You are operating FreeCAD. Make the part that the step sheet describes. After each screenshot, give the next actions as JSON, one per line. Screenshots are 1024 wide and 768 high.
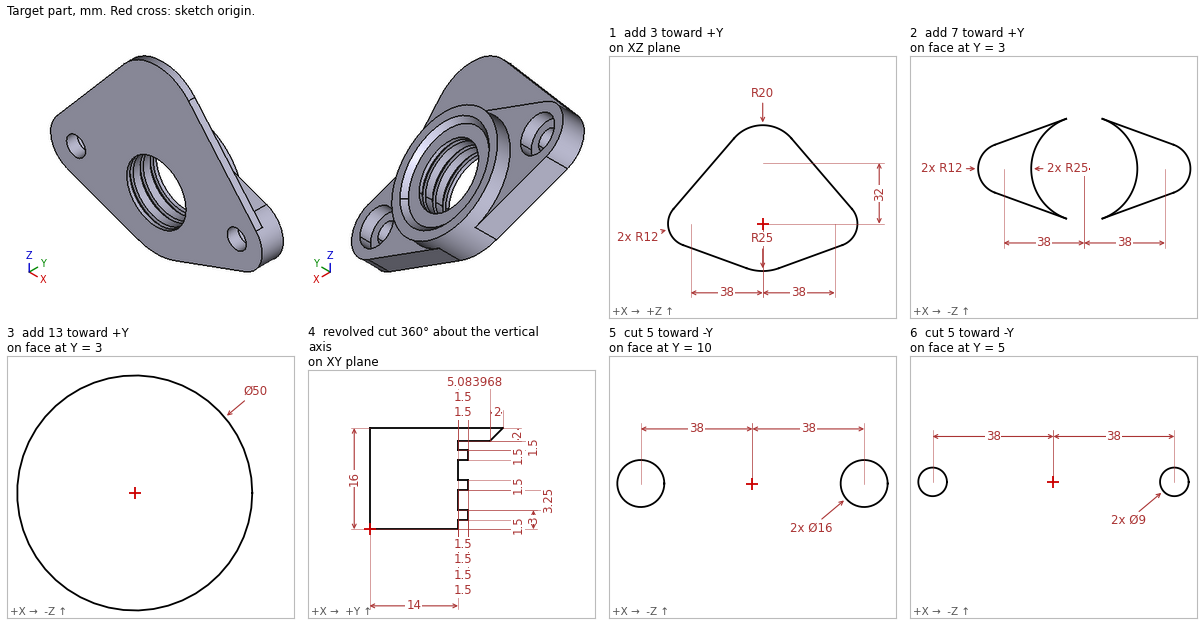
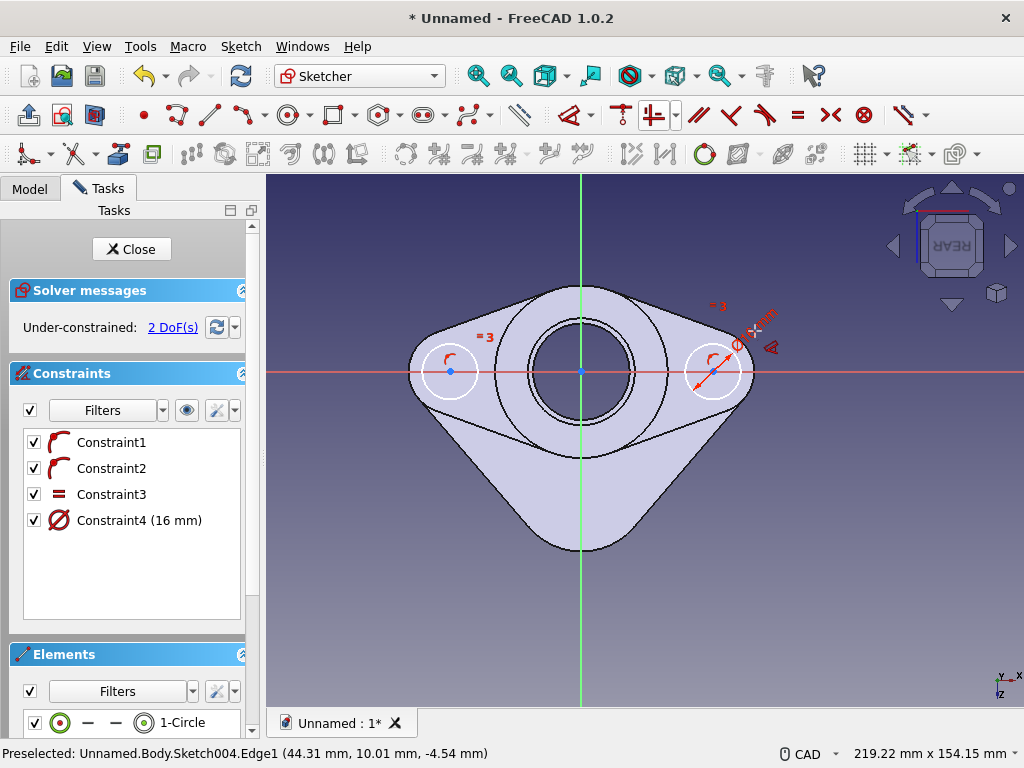
{"action": "left_click", "coordinate": [713, 372]}
{"action": "left_click", "coordinate": [647, 406]}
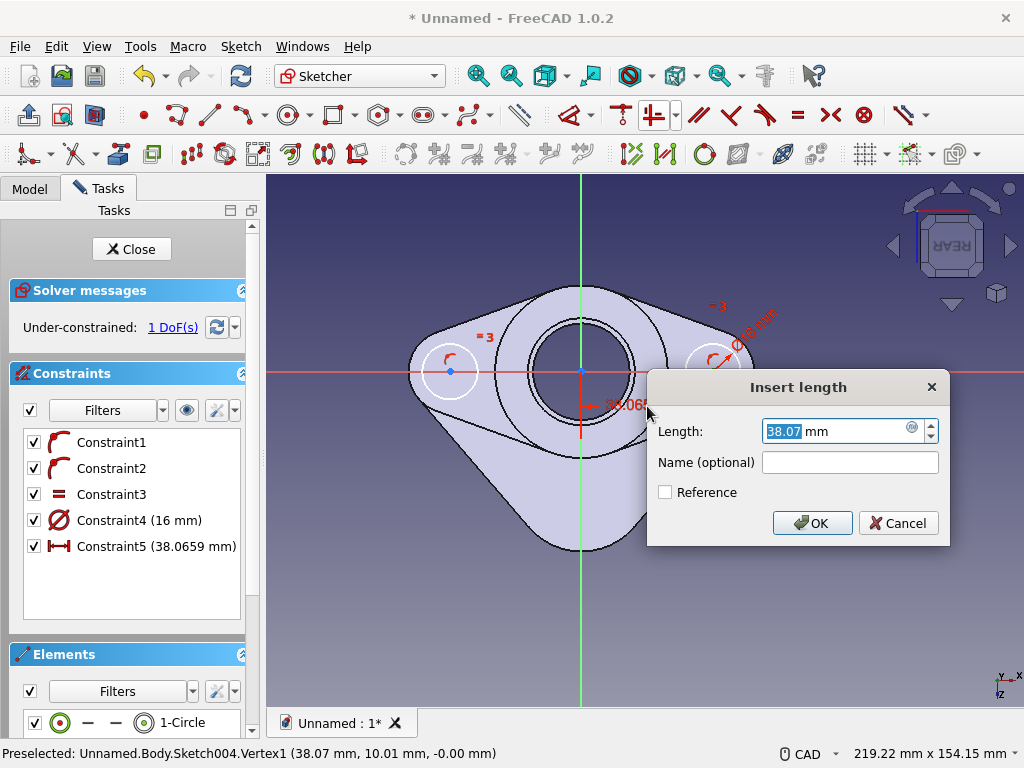
{"action": "type", "text": "38"}
{"action": "key", "text": "Return"}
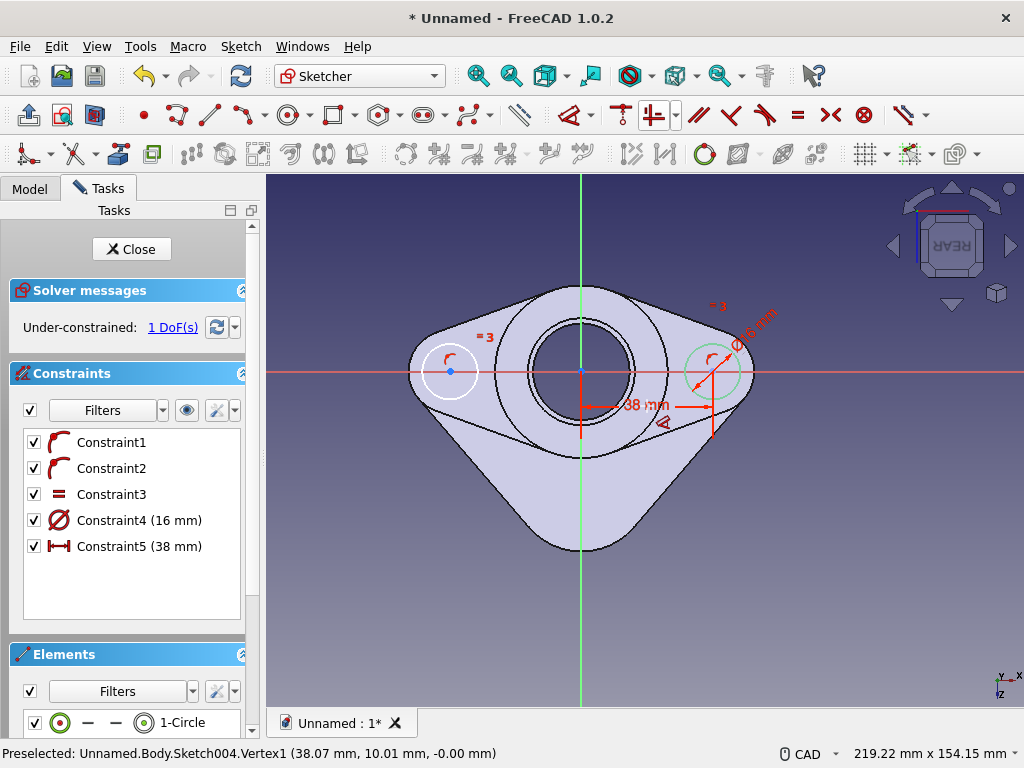
{"action": "left_click", "coordinate": [450, 372]}
{"action": "left_click", "coordinate": [516, 406]}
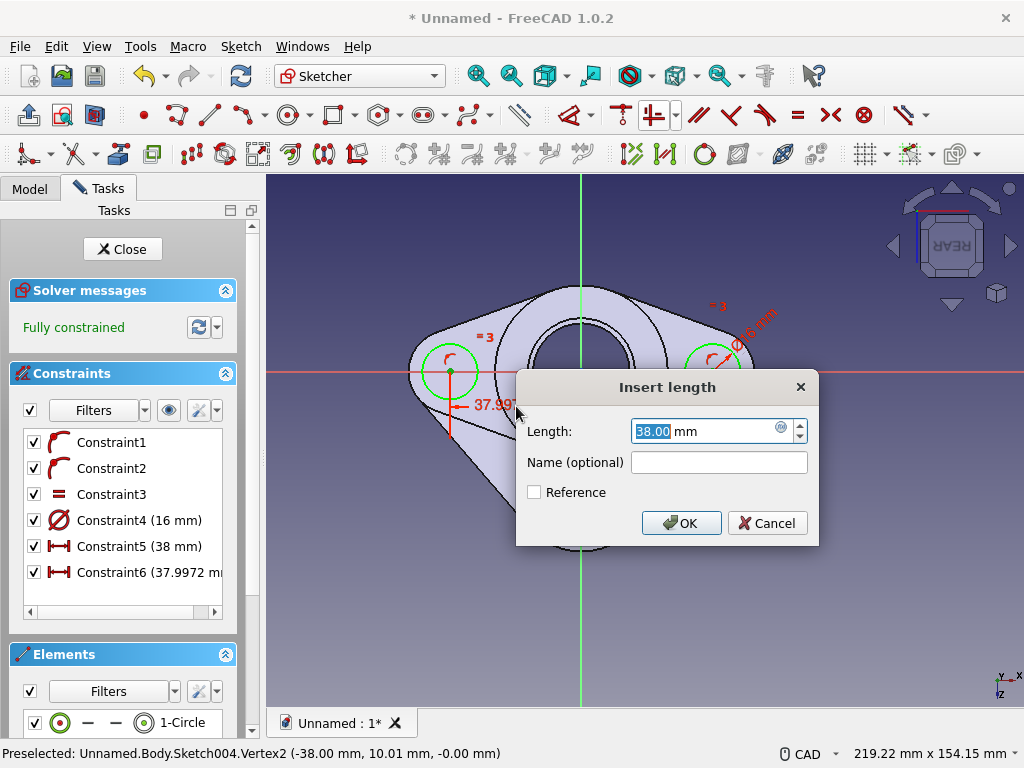
{"action": "type", "text": "38"}
{"action": "key", "text": "Return"}
{"action": "key", "text": "Escape"}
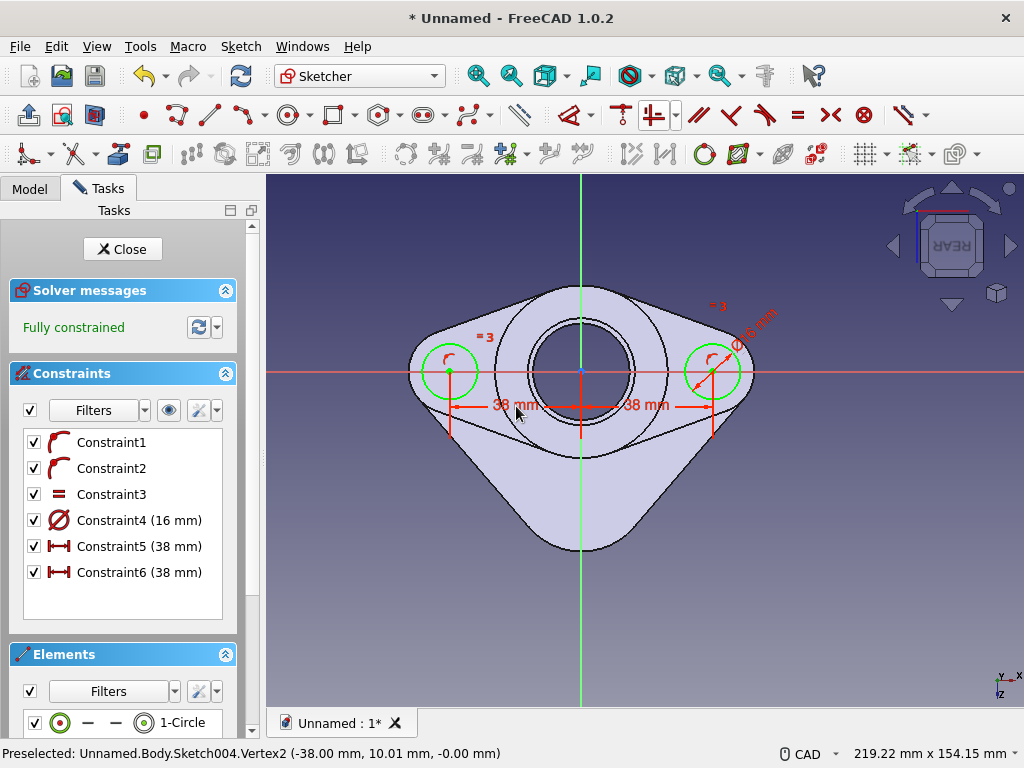
{"action": "left_click", "coordinate": [123, 249]}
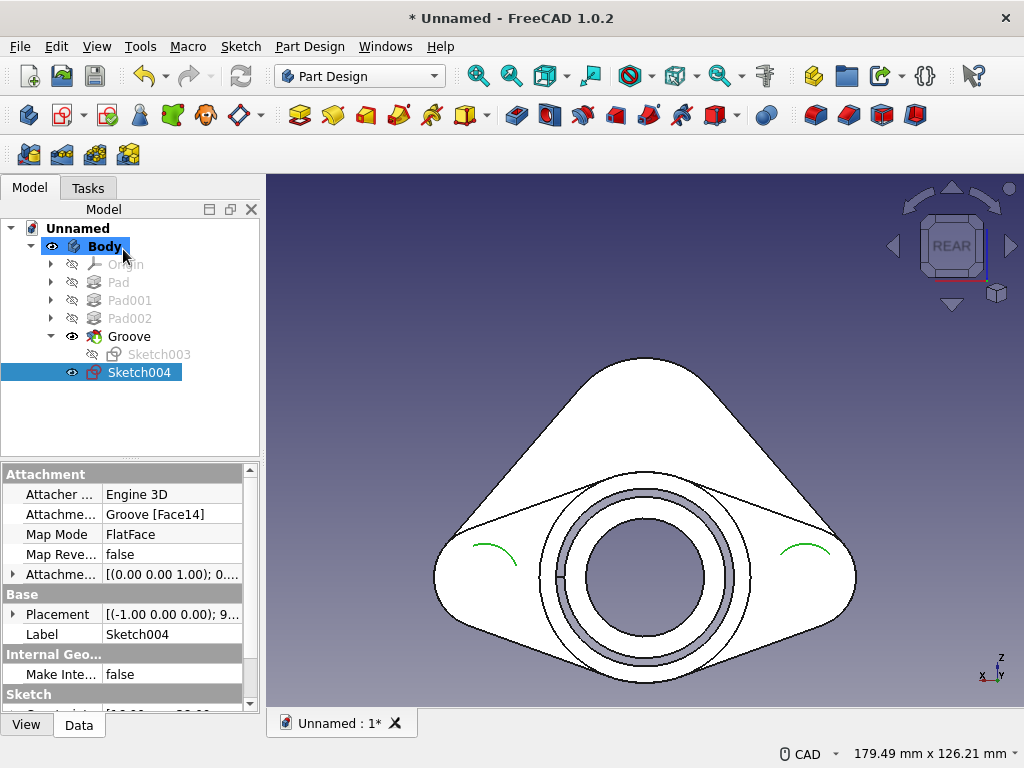
{"action": "left_click", "coordinate": [517, 116]}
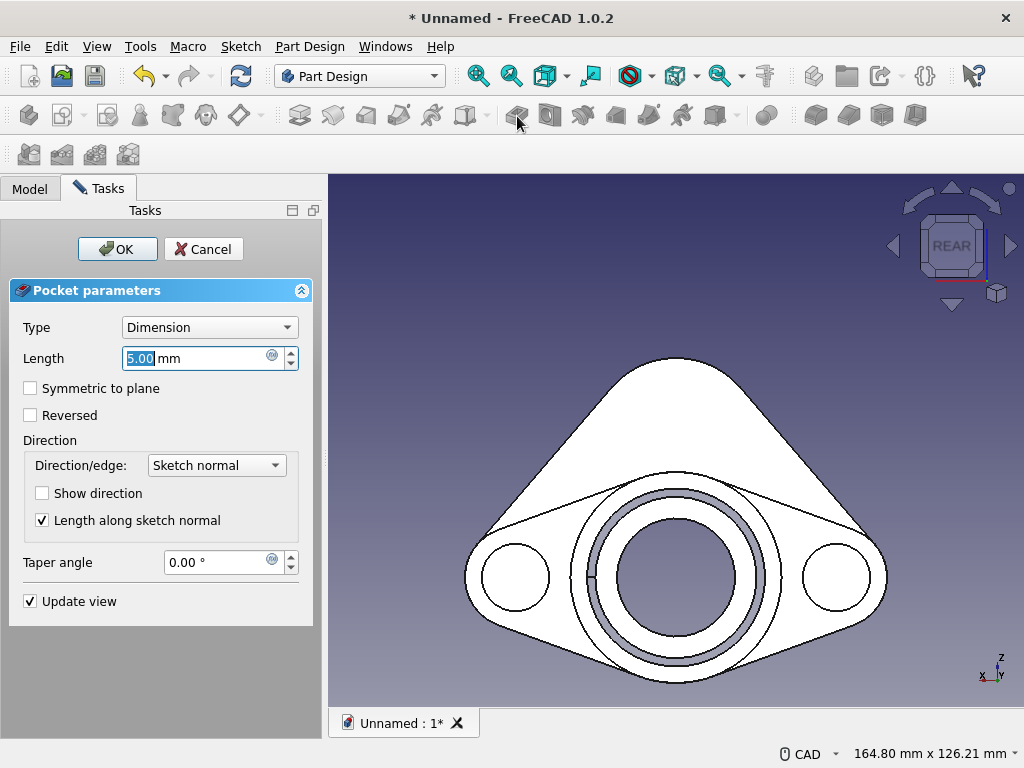
{"action": "type", "text": "5"}
{"action": "key", "text": "Tab"}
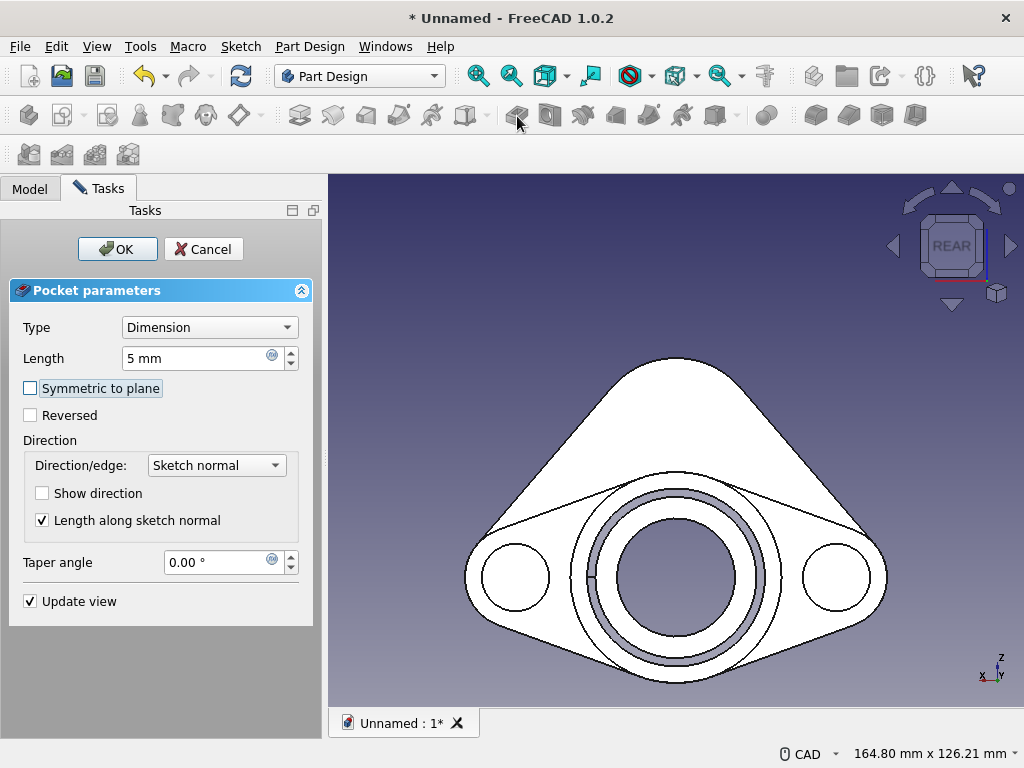
{"action": "left_click", "coordinate": [118, 249]}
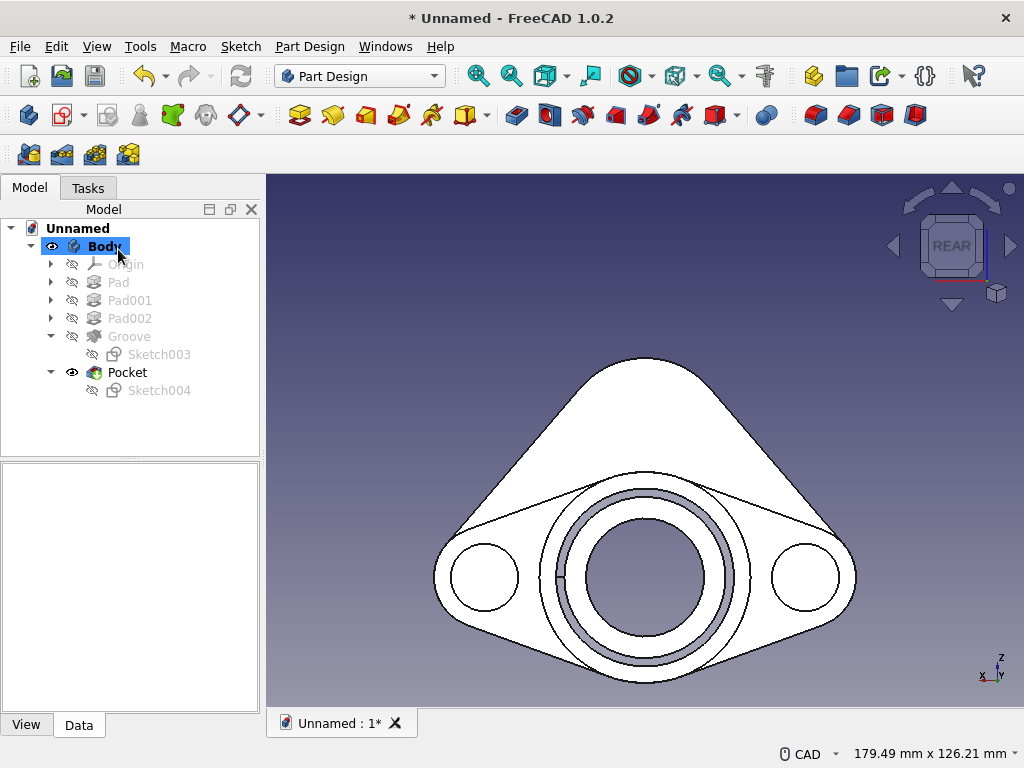
{"action": "left_click", "coordinate": [485, 576]}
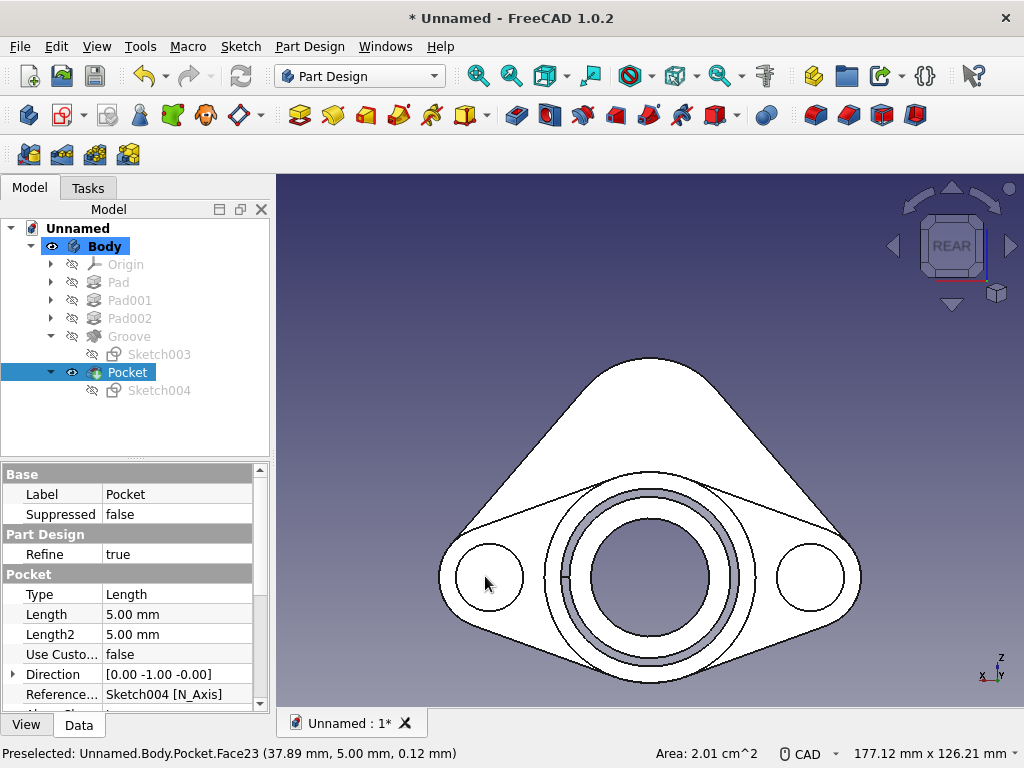
{"action": "left_click", "coordinate": [62, 116]}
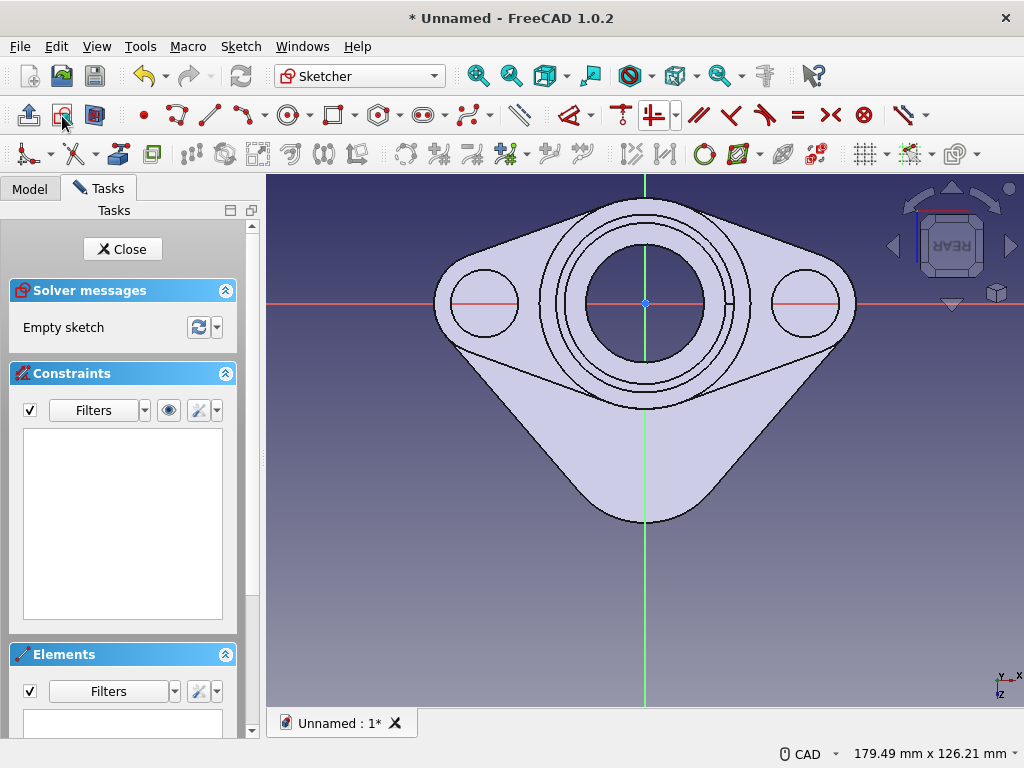
{"action": "left_click", "coordinate": [288, 116]}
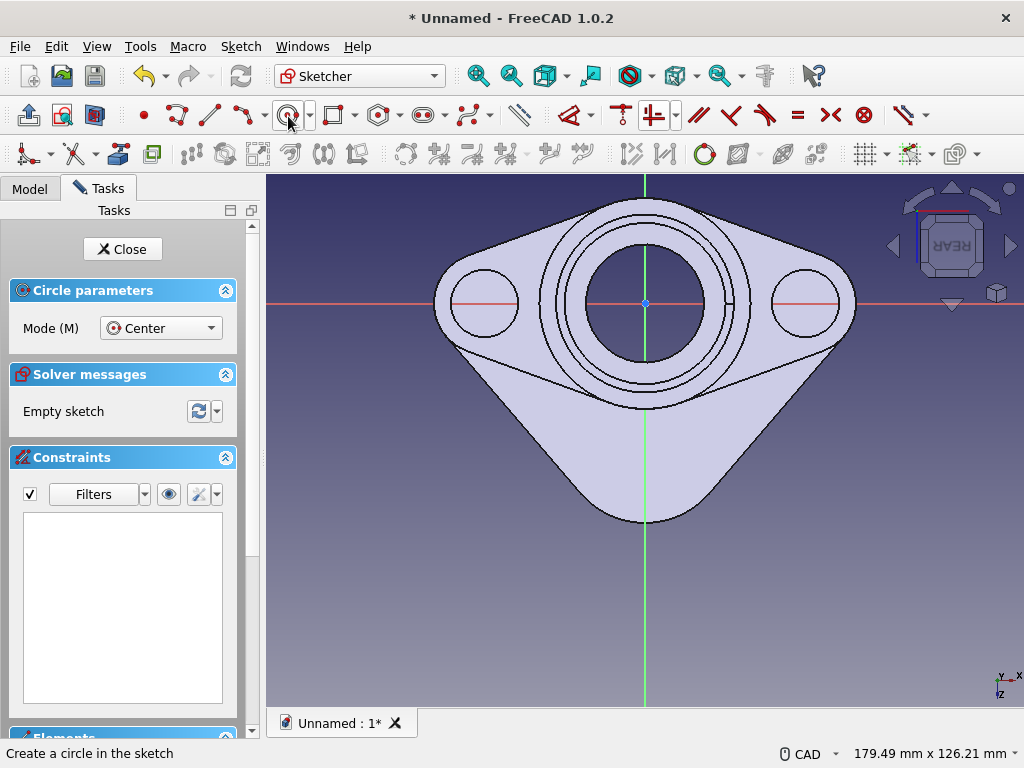
{"action": "left_click", "coordinate": [805, 304]}
{"action": "left_click", "coordinate": [812, 286]}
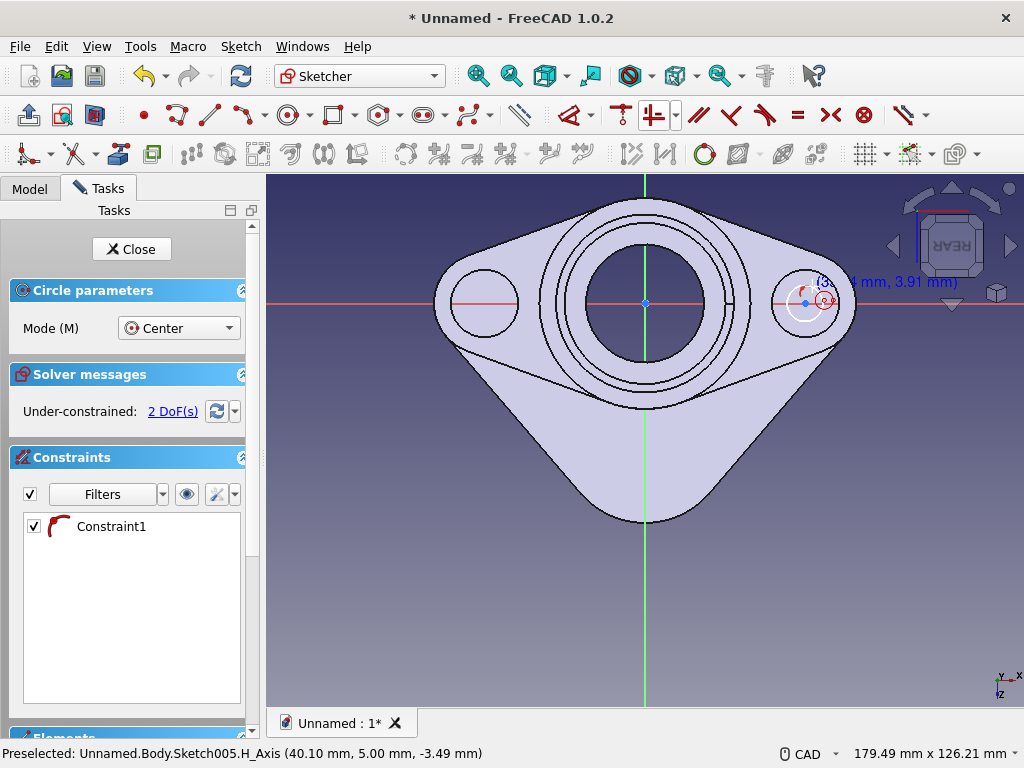
{"action": "left_click", "coordinate": [485, 304]}
{"action": "left_click", "coordinate": [491, 286]}
{"action": "key", "text": "Escape"}